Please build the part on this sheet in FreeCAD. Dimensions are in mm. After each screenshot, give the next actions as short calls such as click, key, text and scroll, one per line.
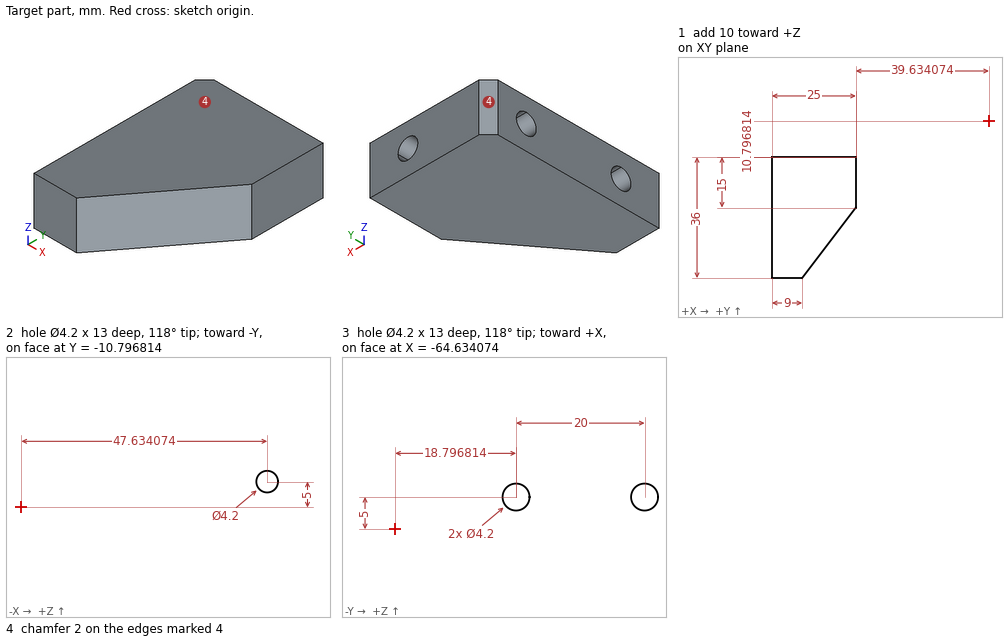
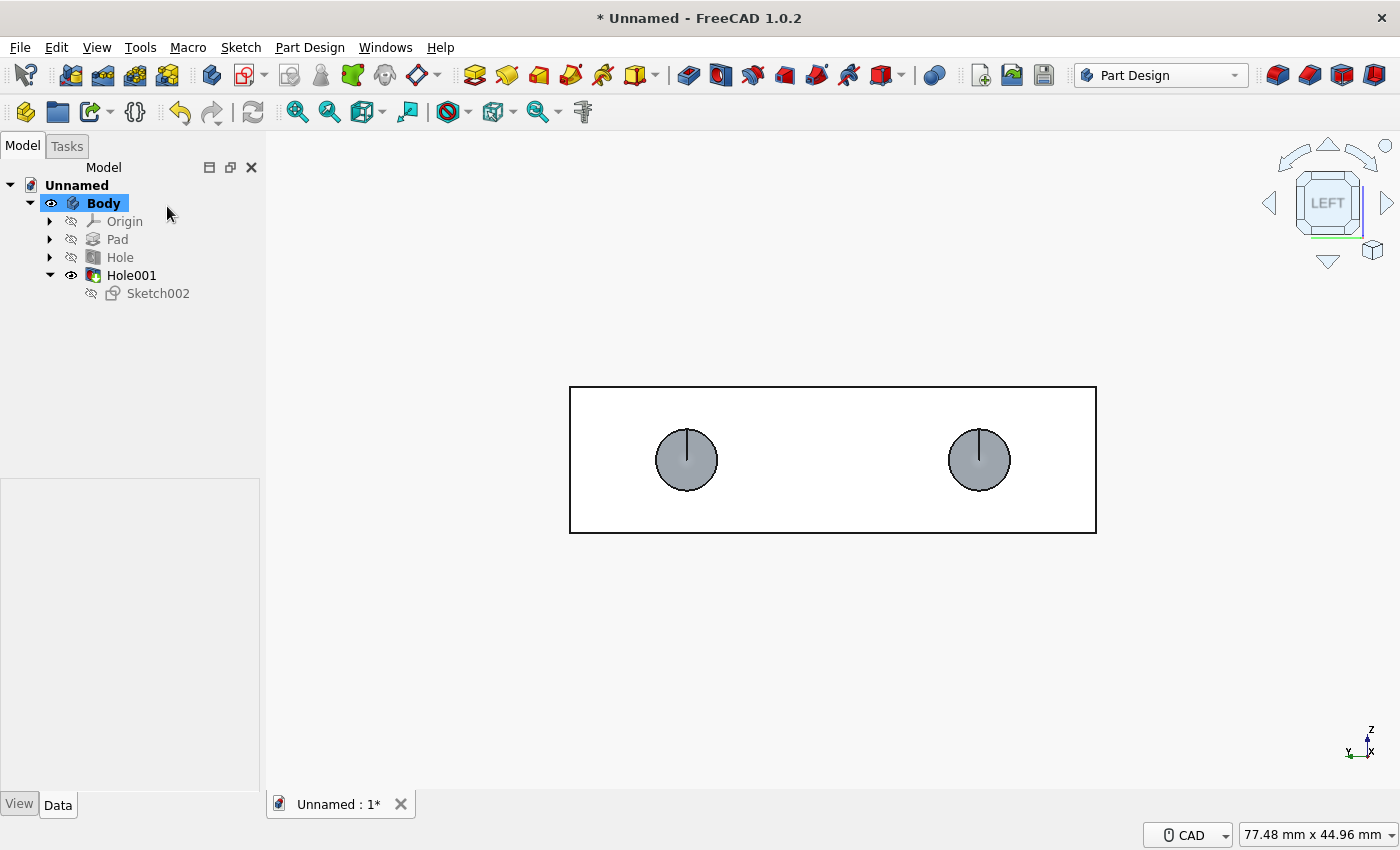
click(570, 459)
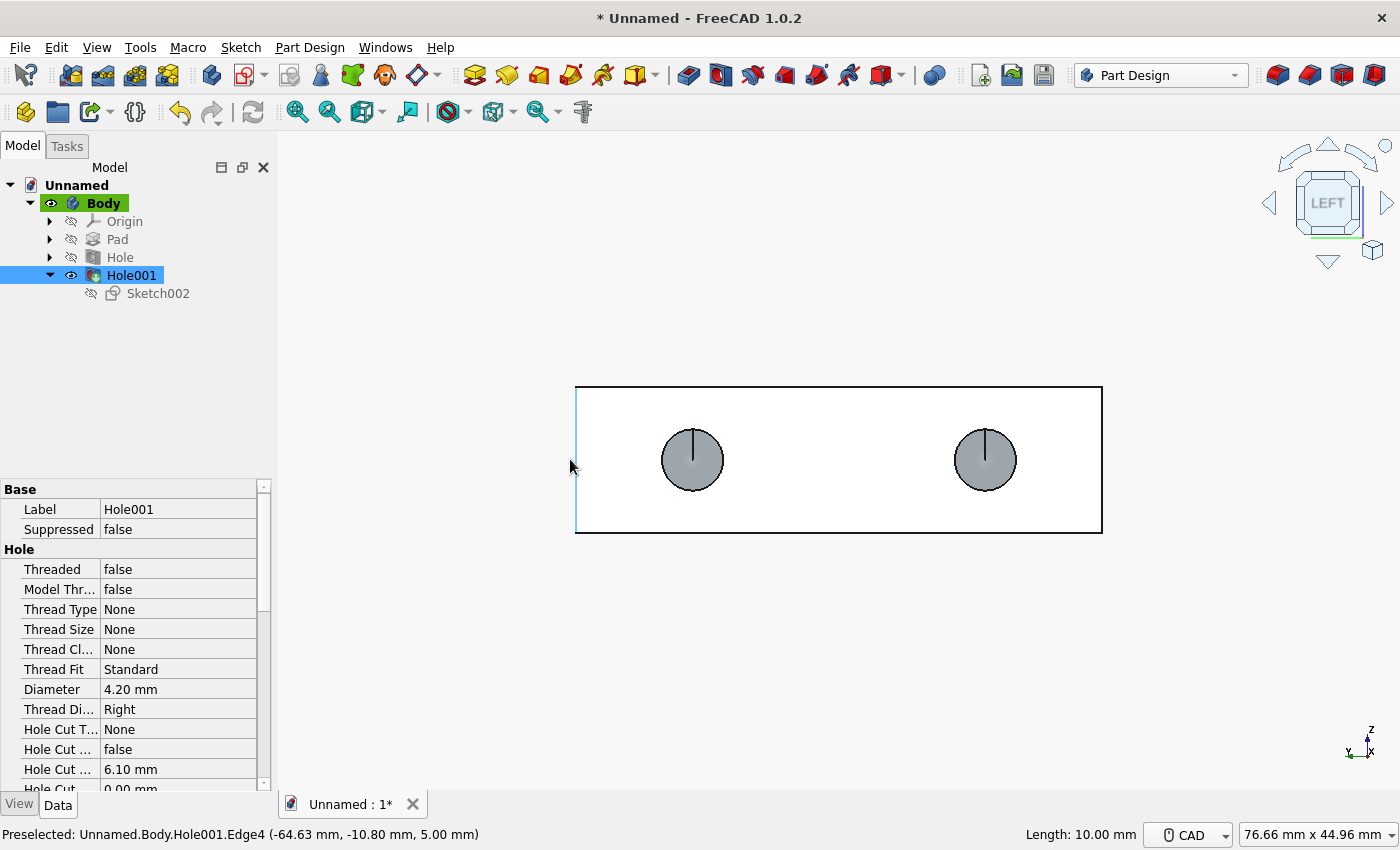
click(1310, 76)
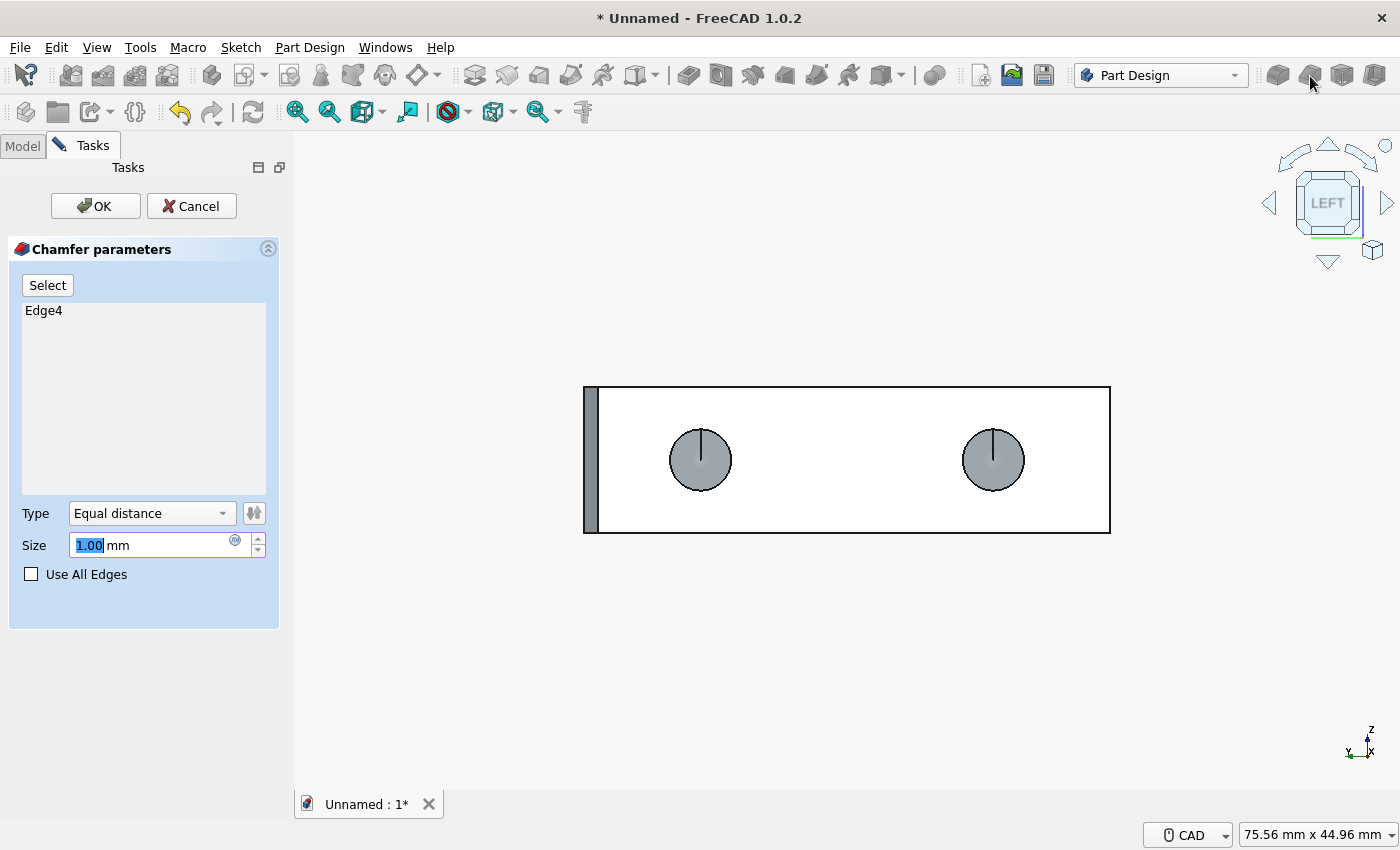
text(2)
key(Tab)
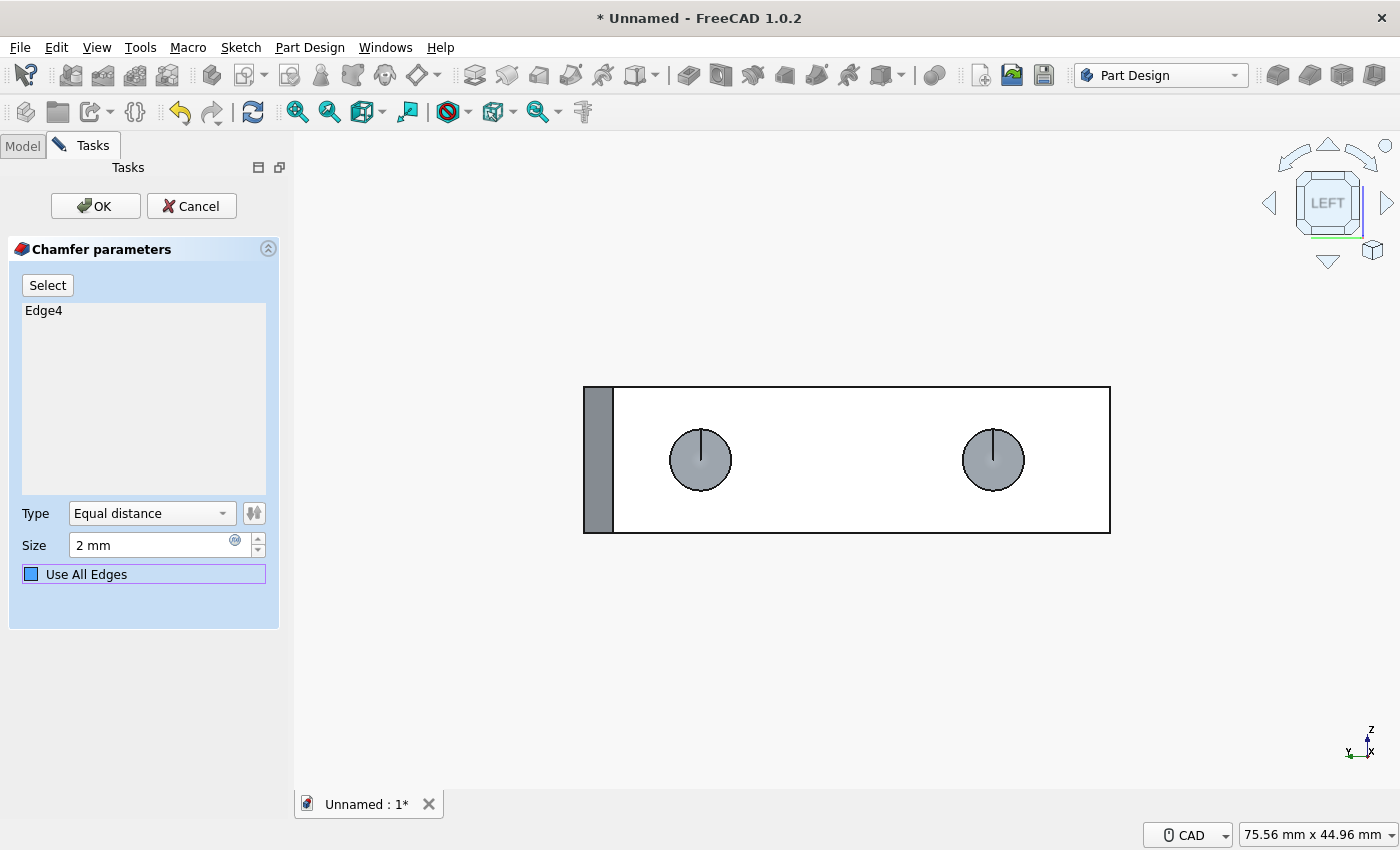
click(96, 206)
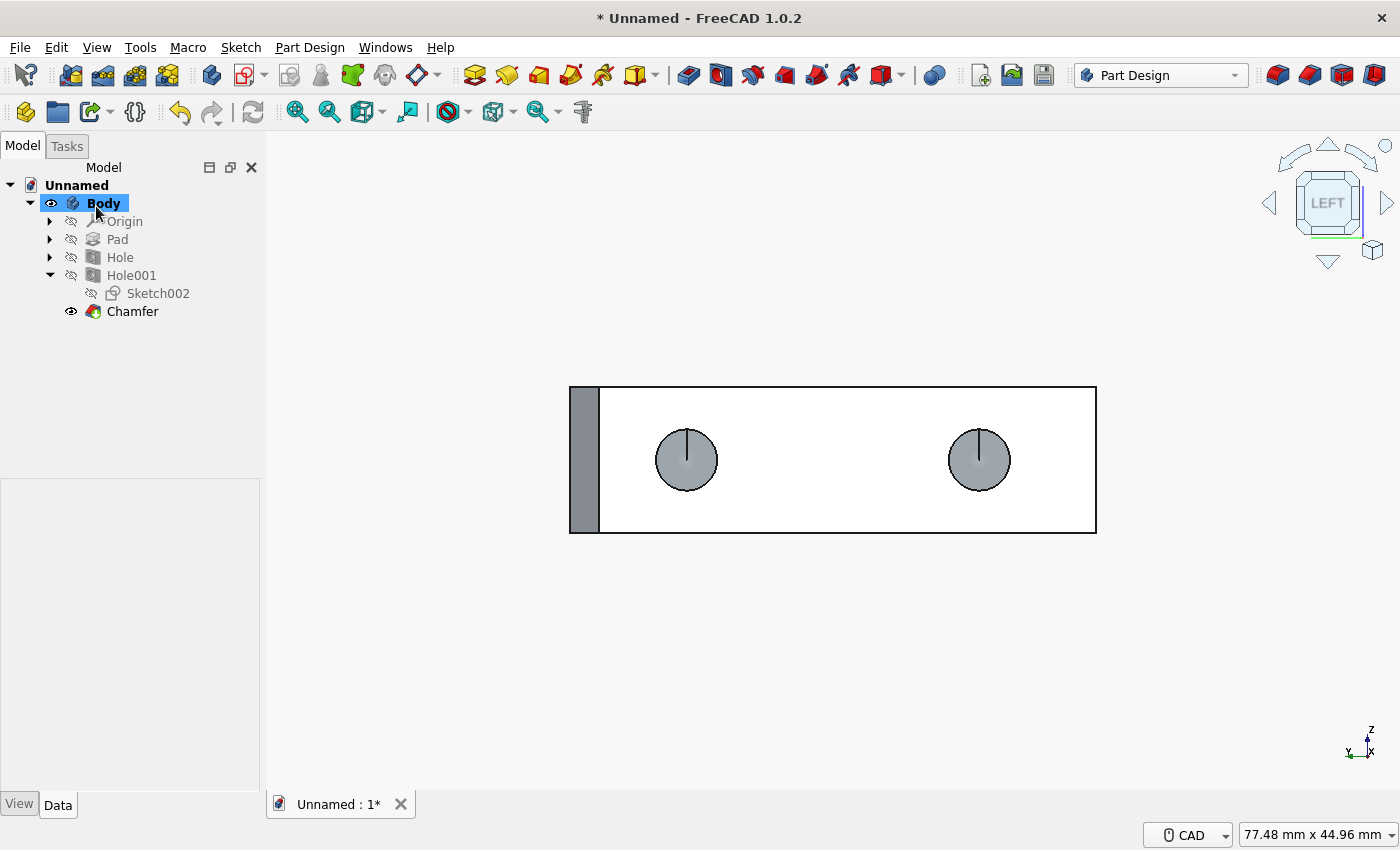
key(0)